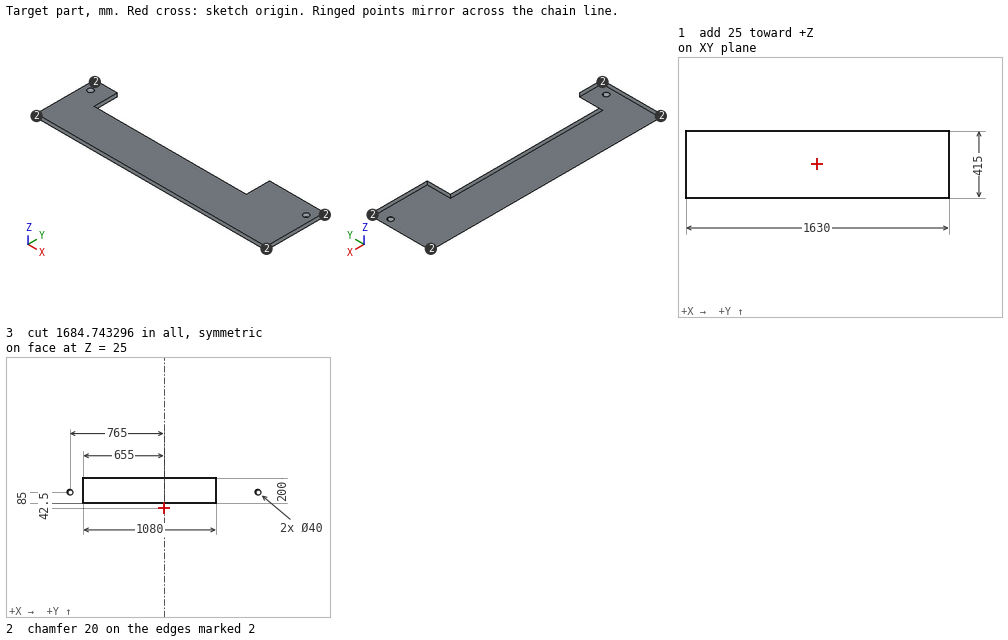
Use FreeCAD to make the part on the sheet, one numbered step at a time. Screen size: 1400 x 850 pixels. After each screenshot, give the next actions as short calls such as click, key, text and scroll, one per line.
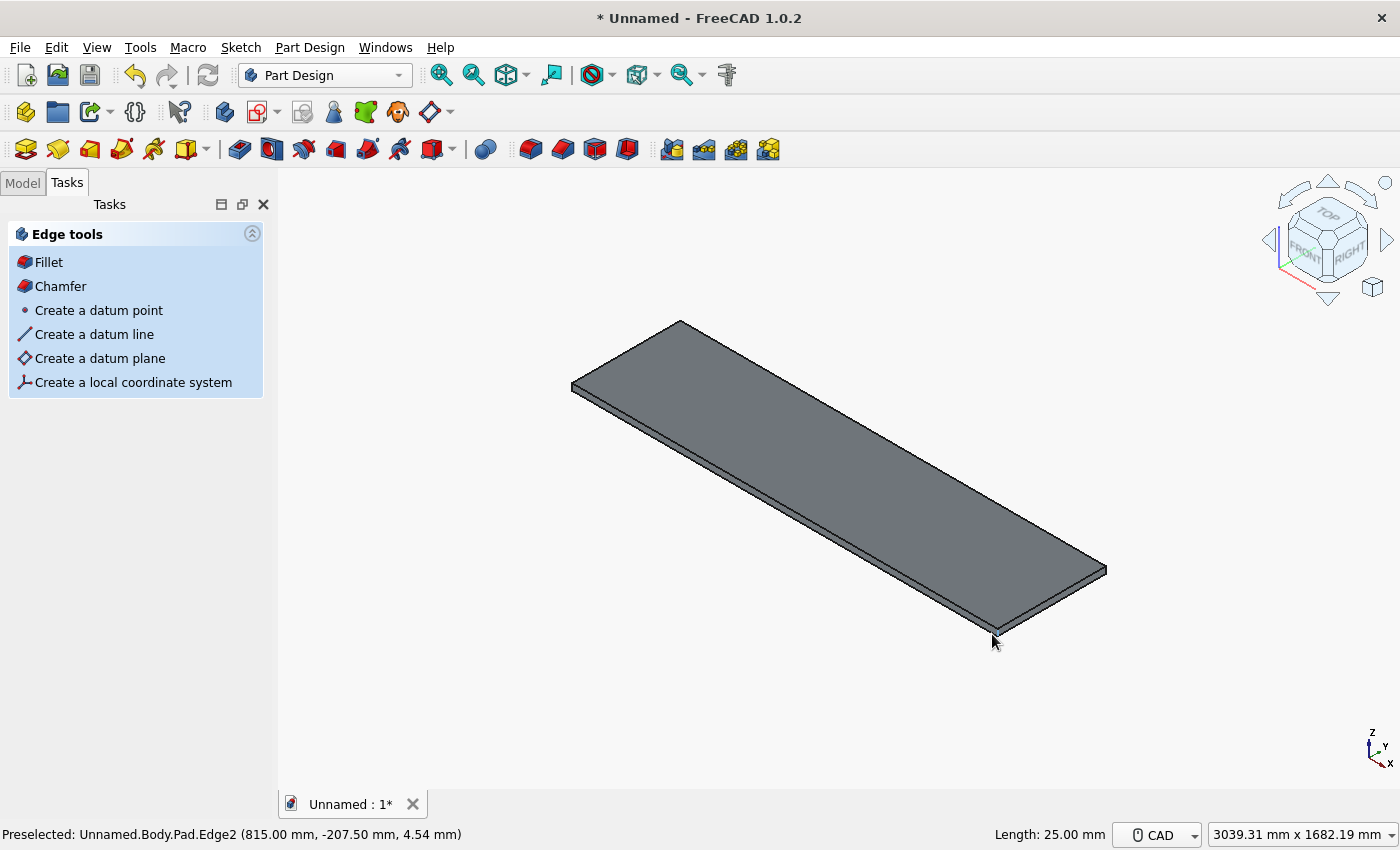
scroll(680, 323, up, 8)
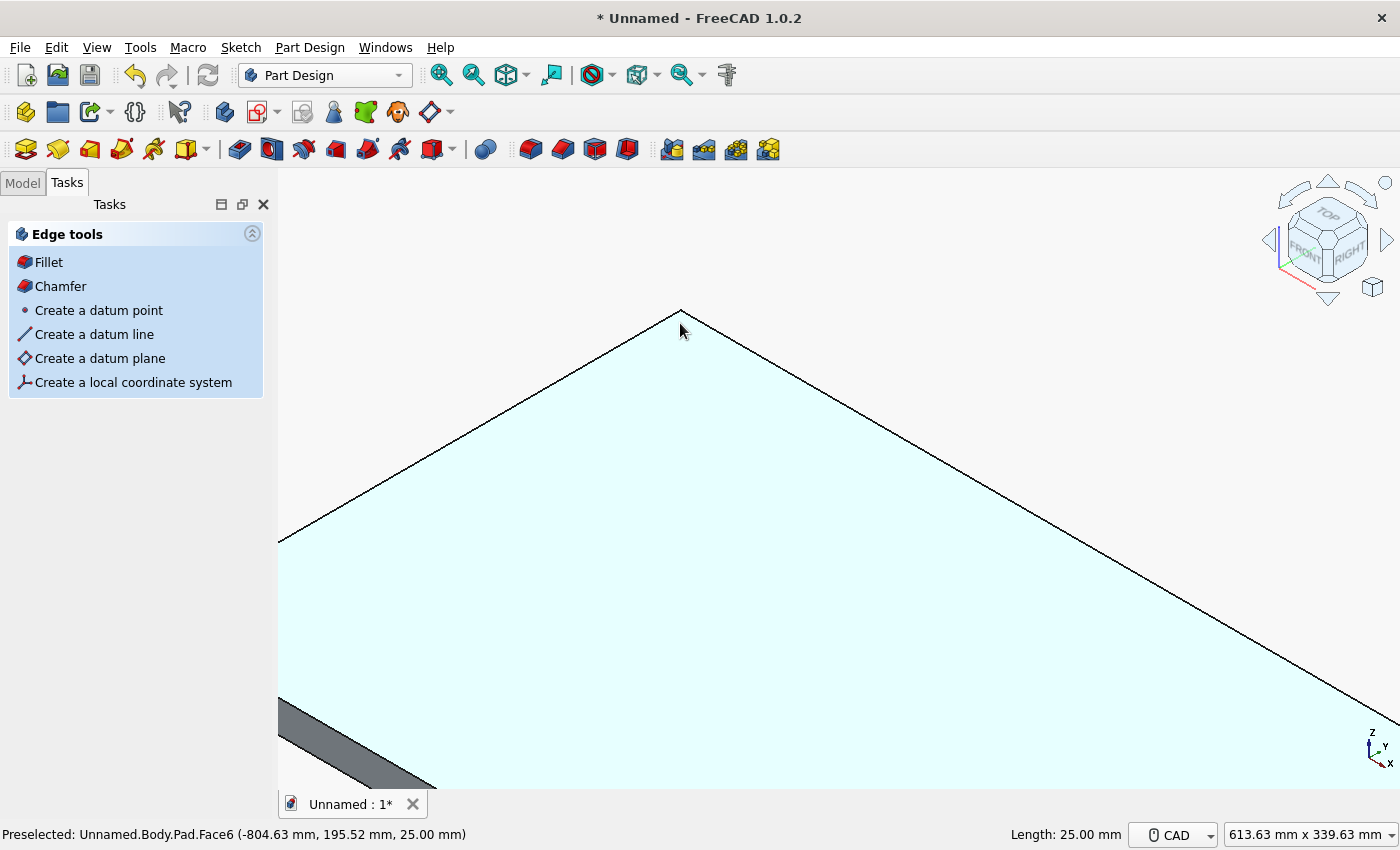
click(442, 76)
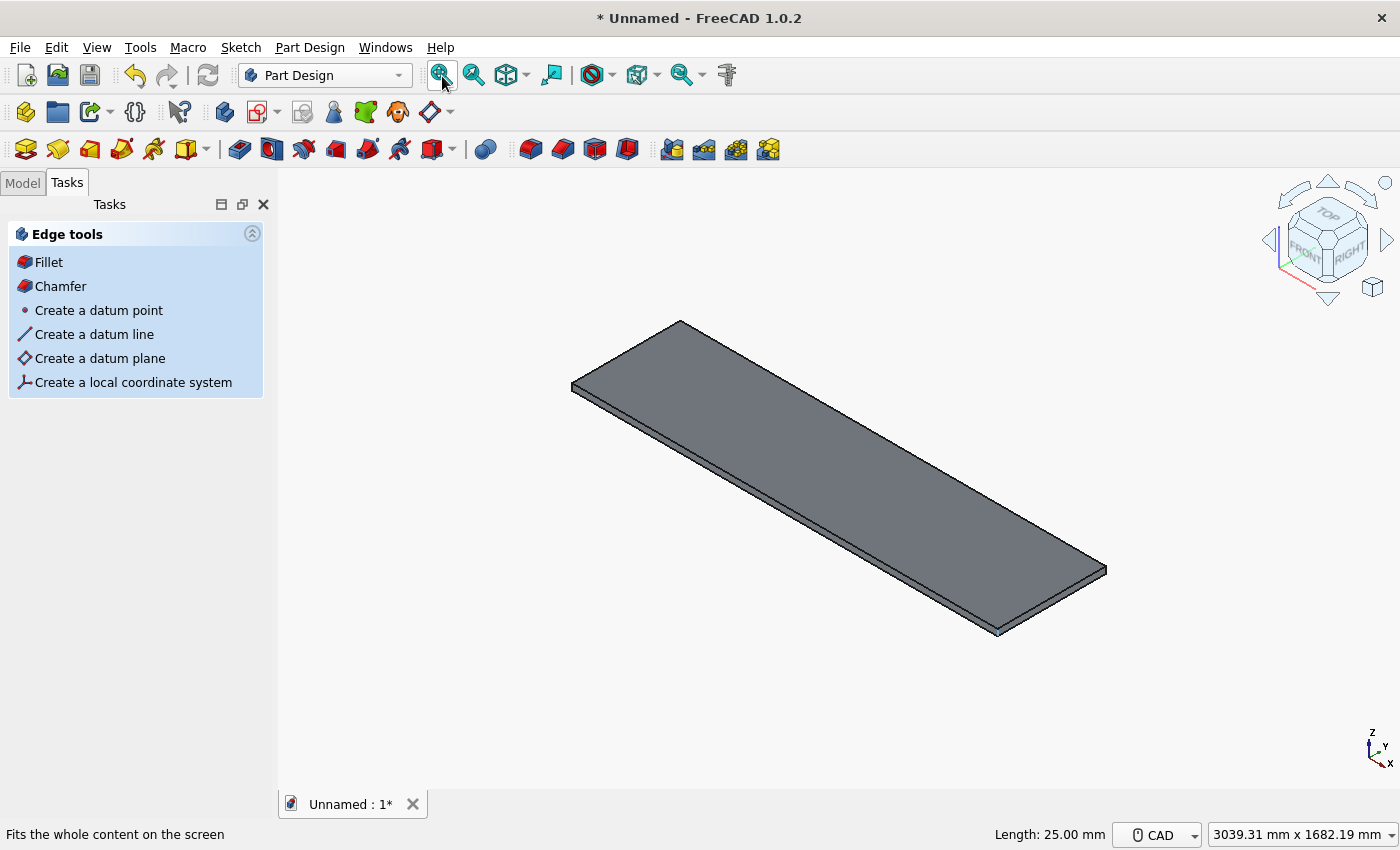
key(2)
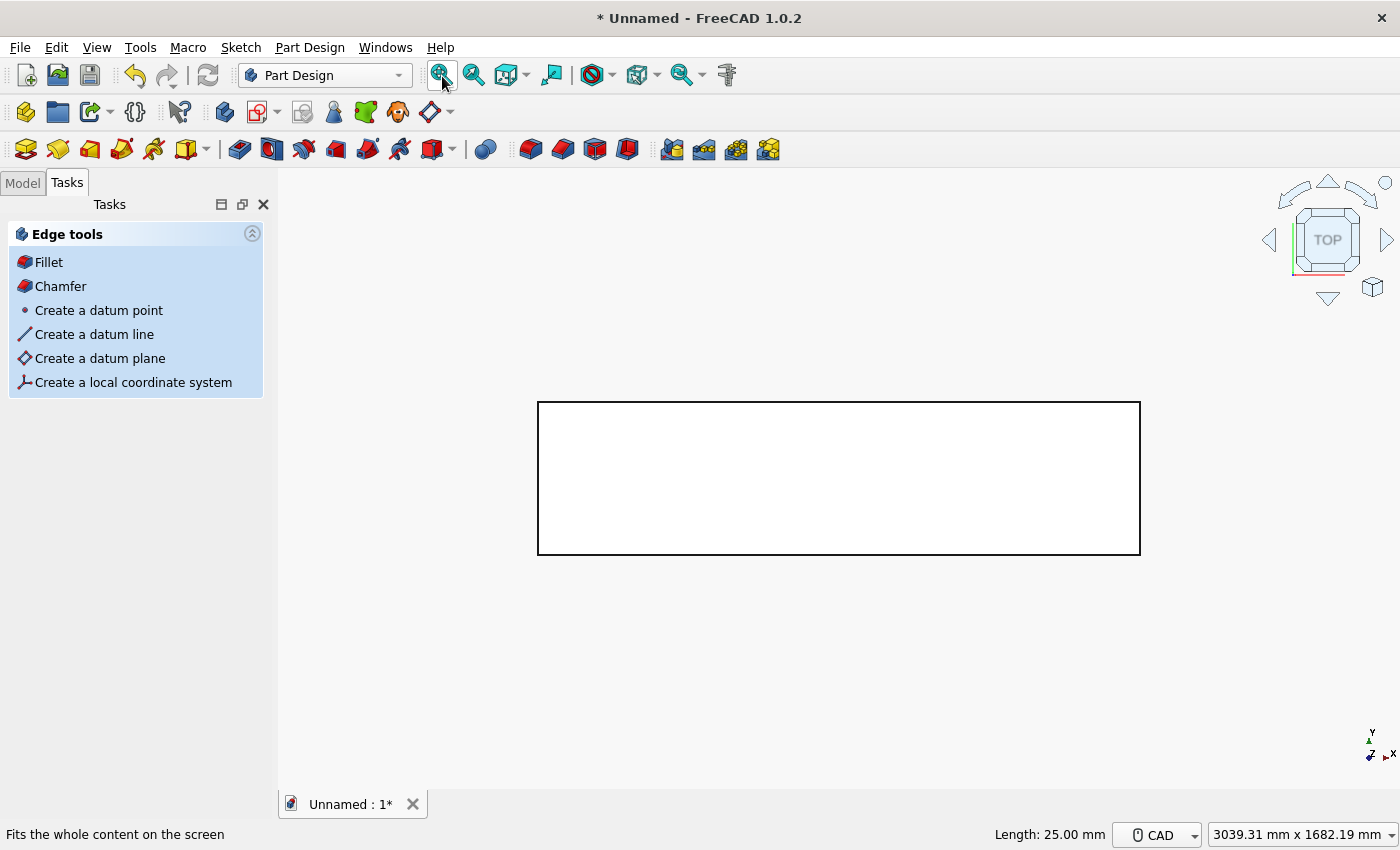
scroll(538, 401, up, 8)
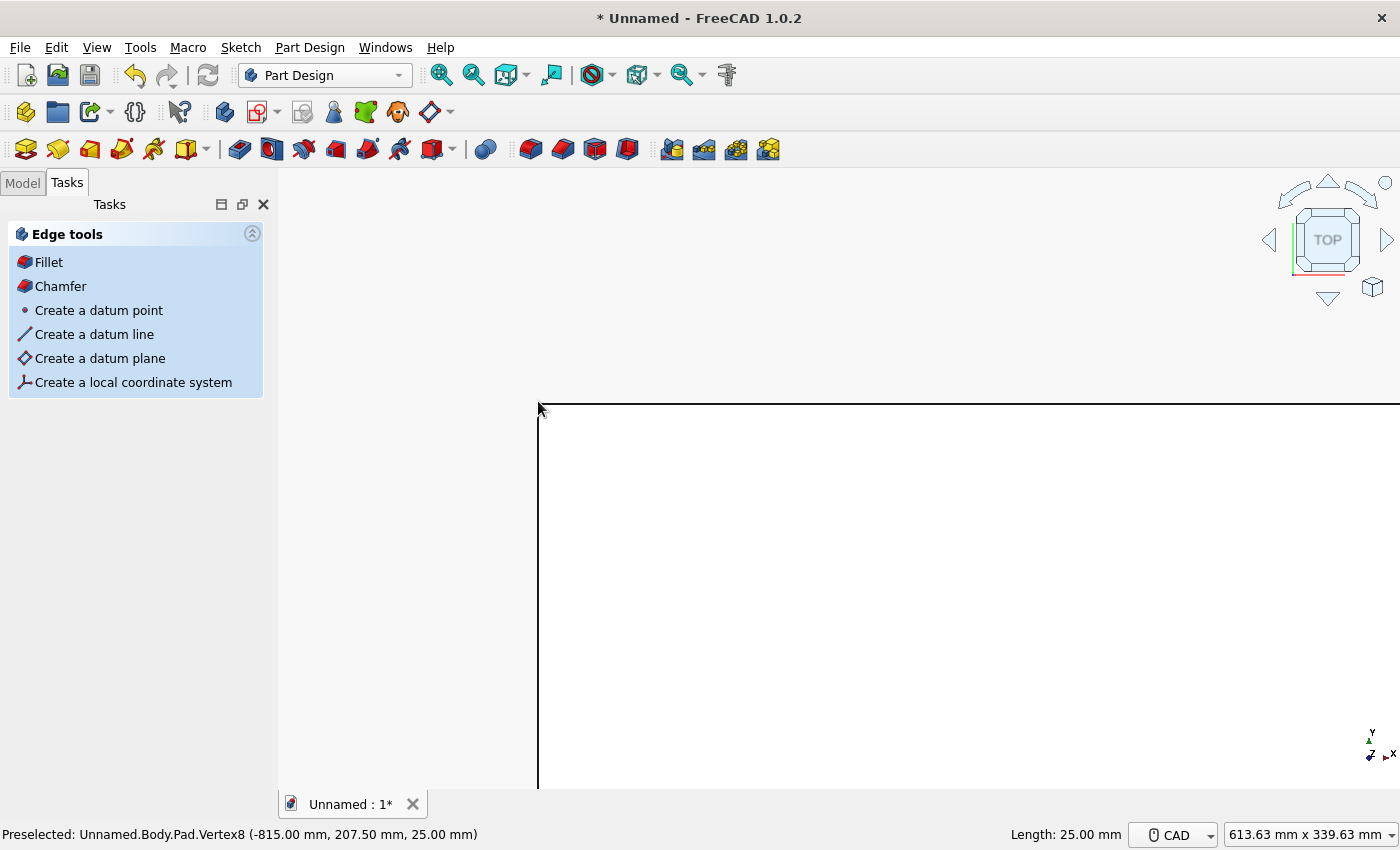
click(442, 76)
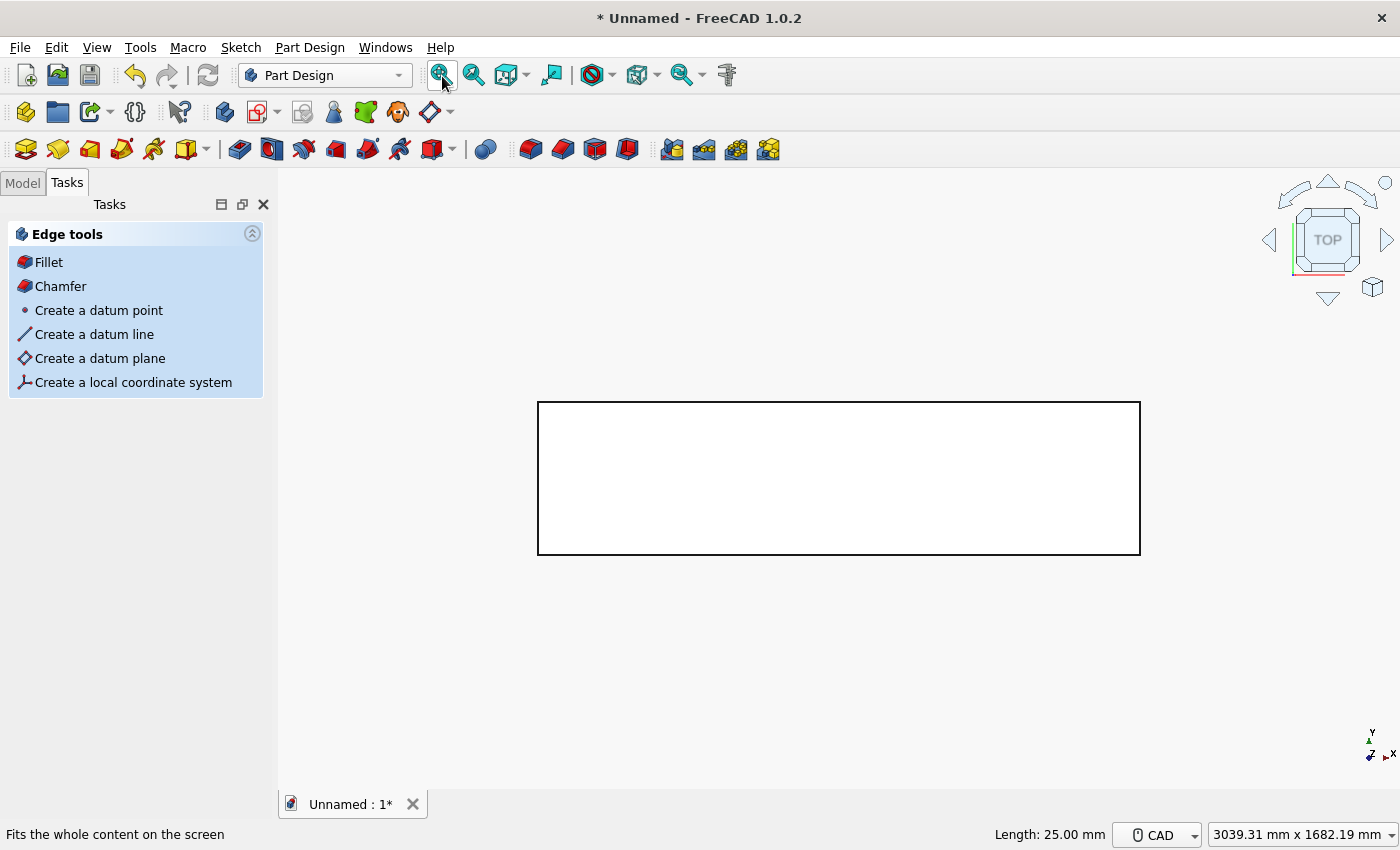
key(1)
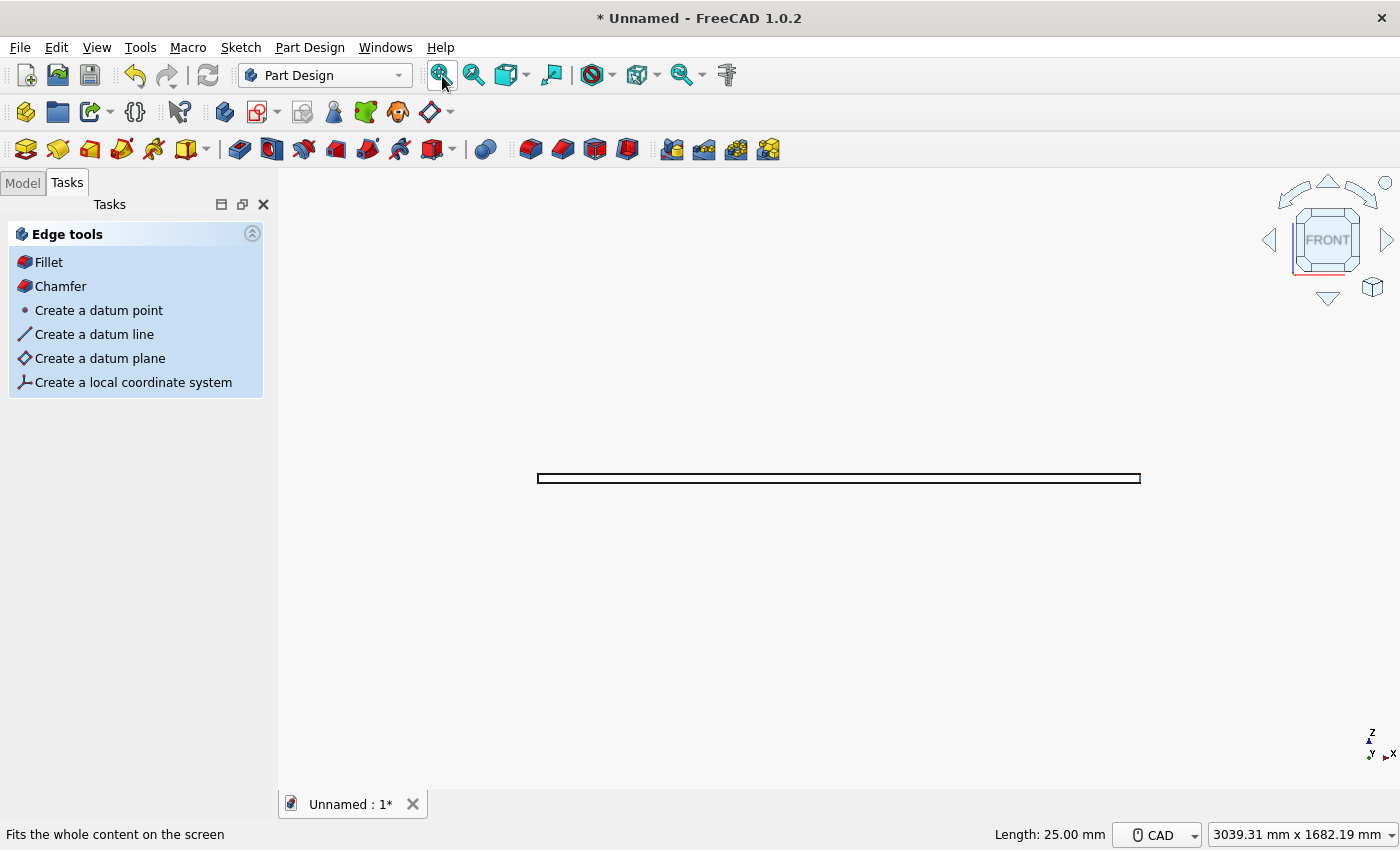
scroll(538, 478, up, 8)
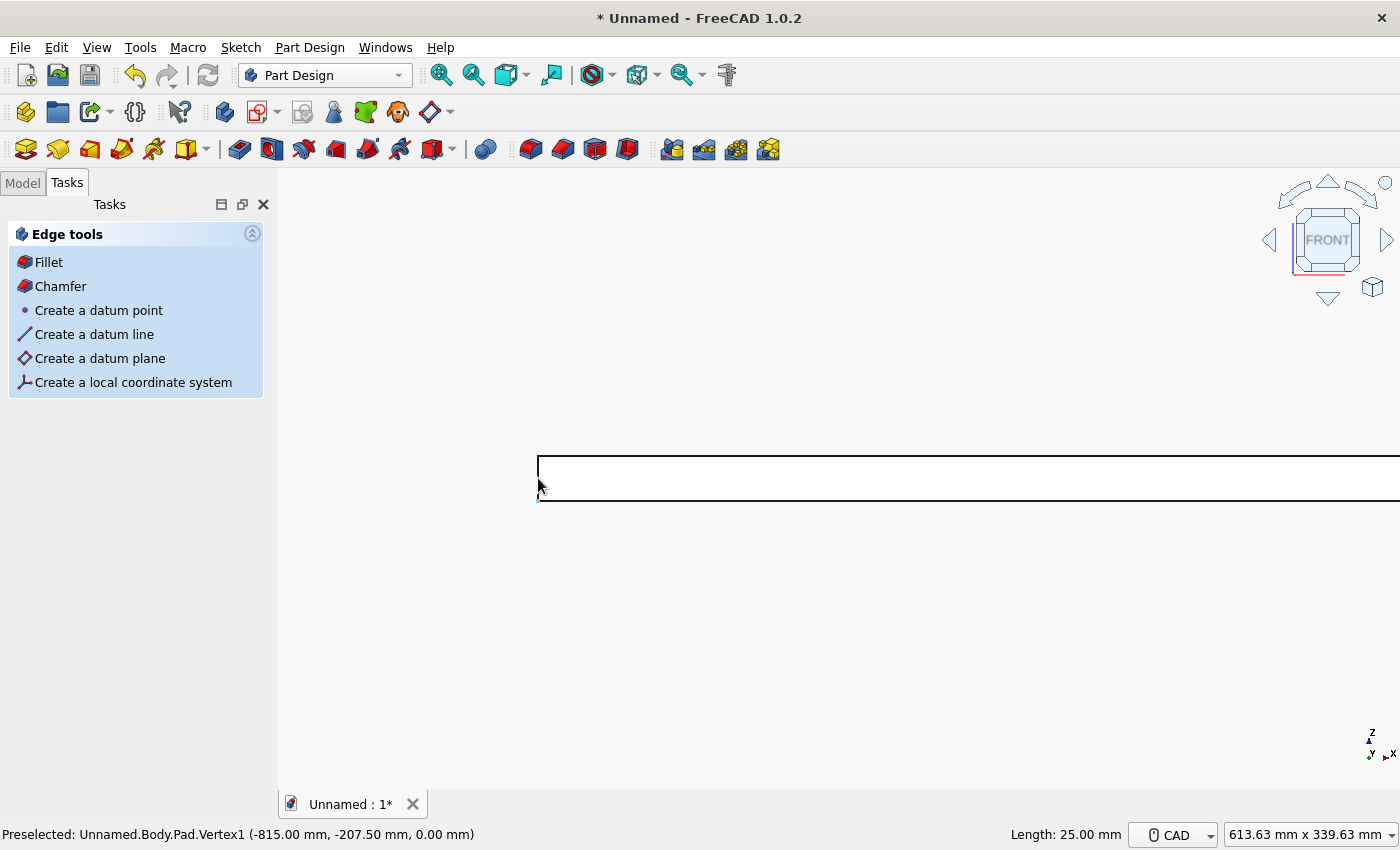
click(538, 478, ctrl)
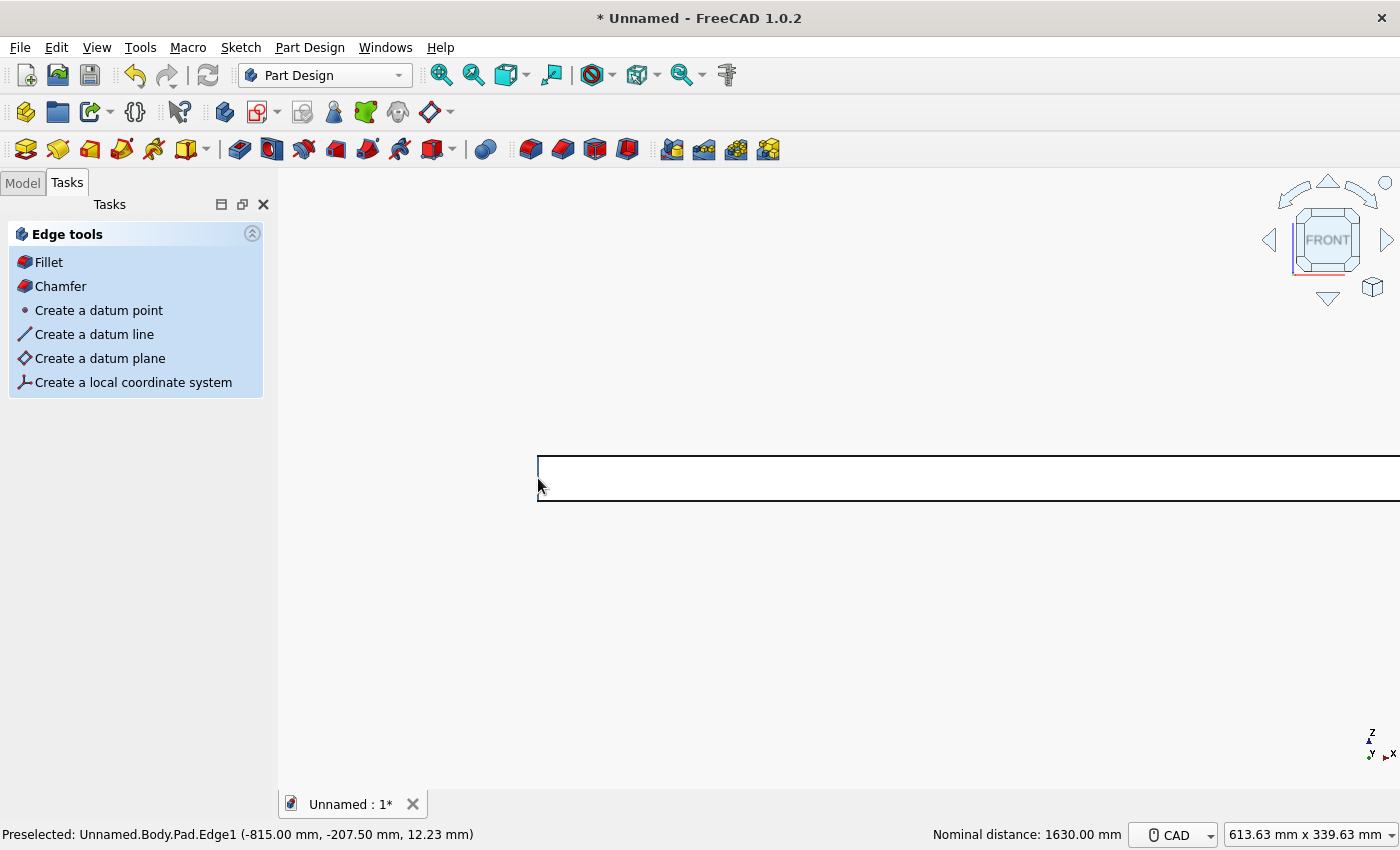
click(442, 76)